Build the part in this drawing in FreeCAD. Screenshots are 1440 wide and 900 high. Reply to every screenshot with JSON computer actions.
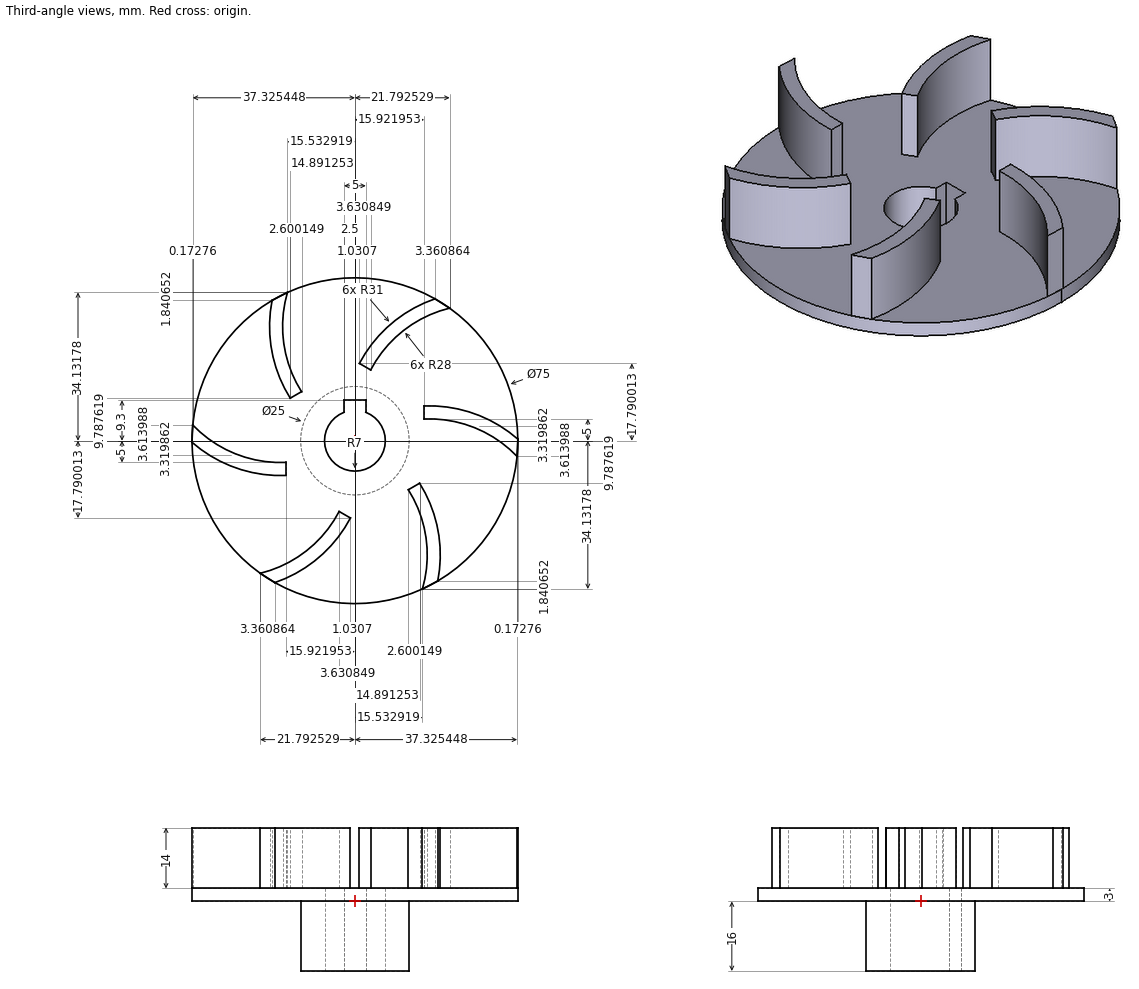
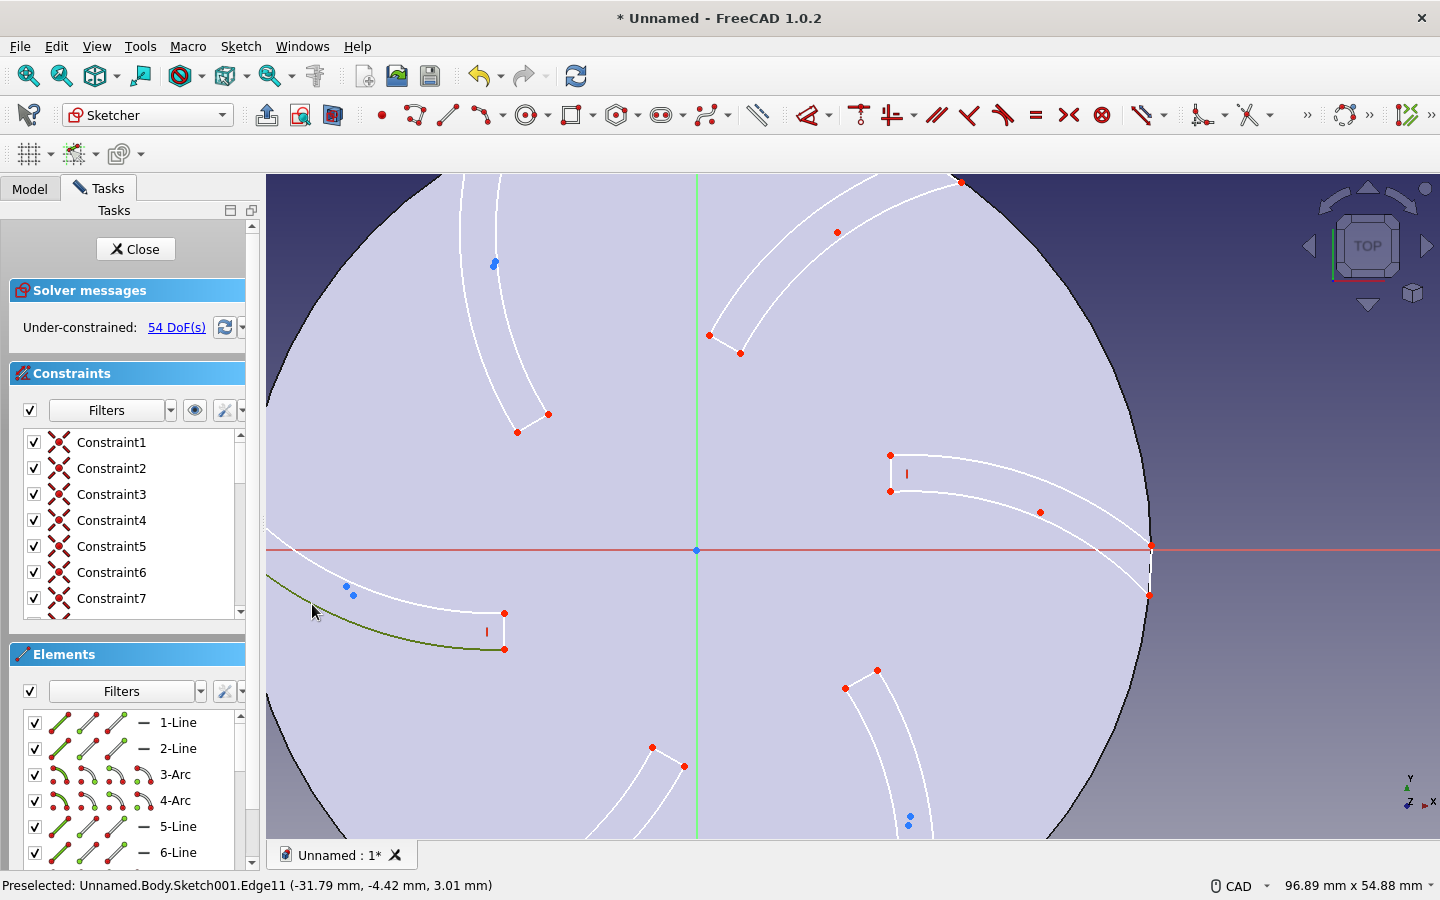
{"action": "scroll", "coordinate": [311, 561], "scroll_direction": "up", "scroll_amount": 2}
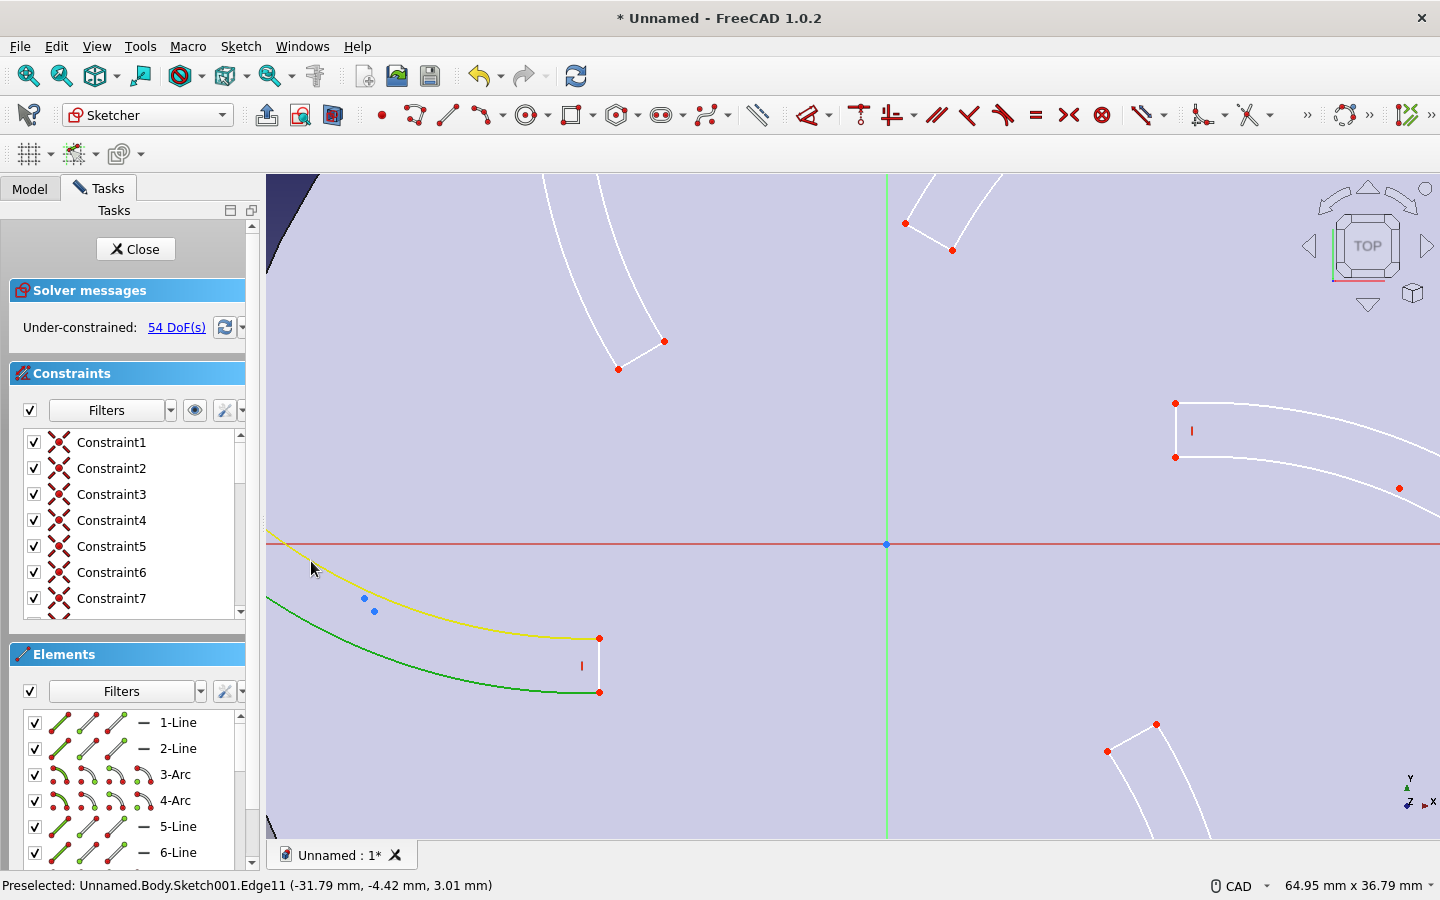
{"action": "left_click", "coordinate": [311, 561]}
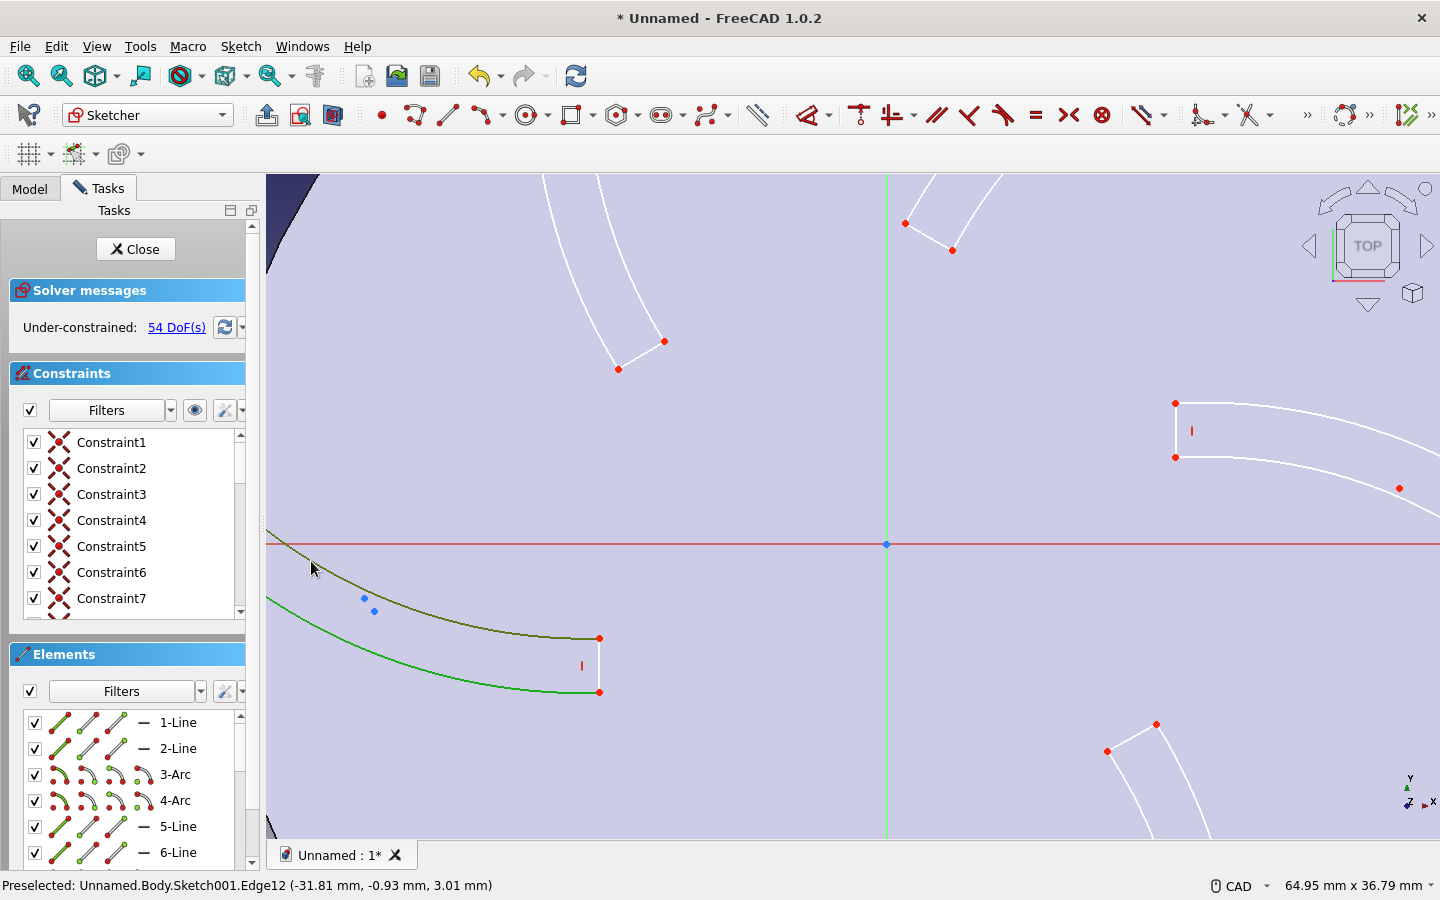
{"action": "left_click", "coordinate": [859, 116]}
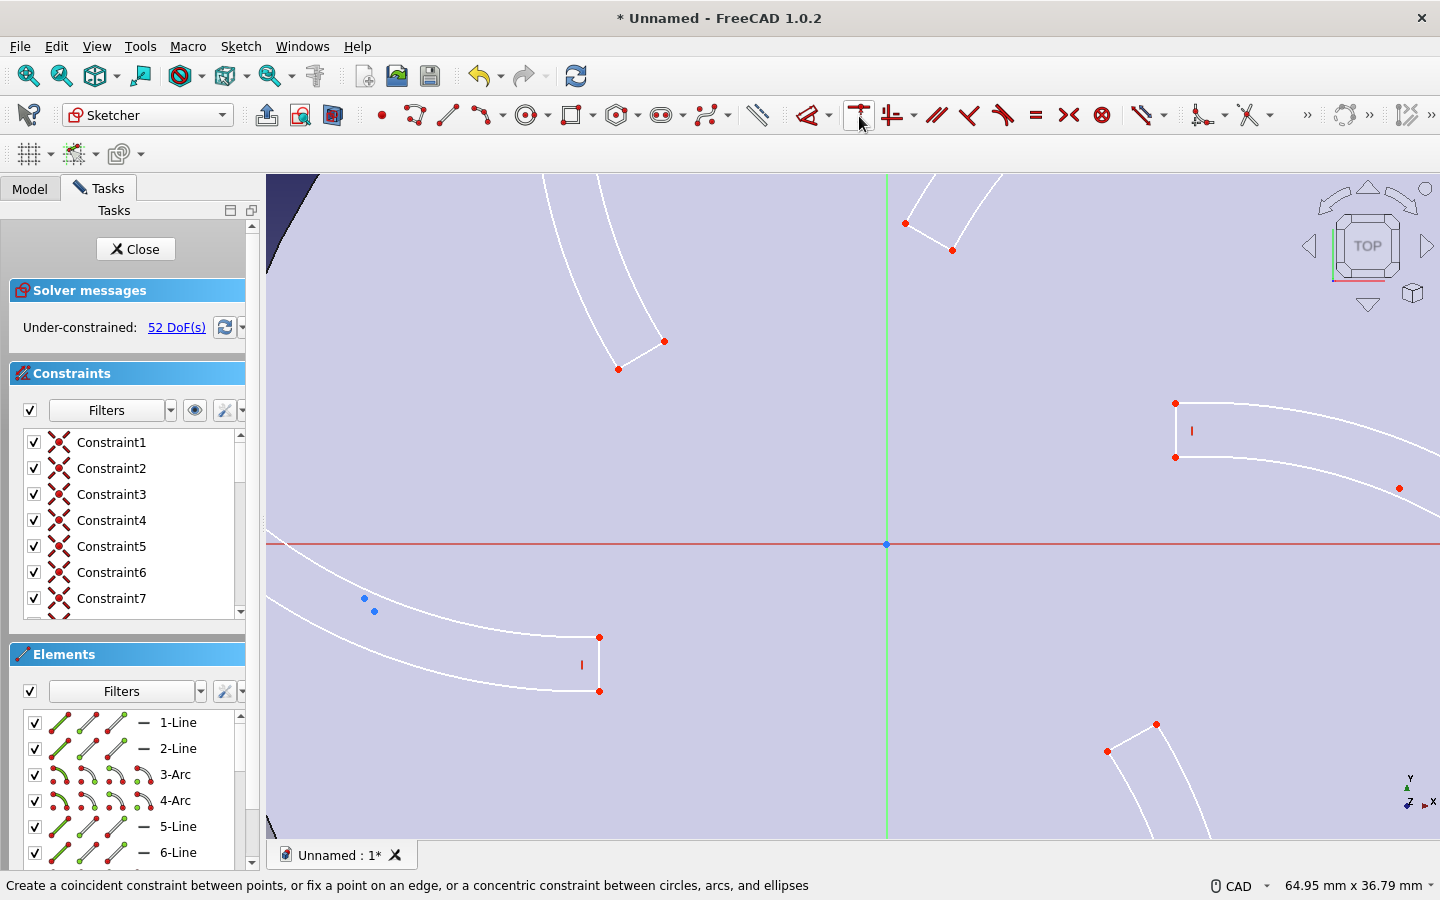
{"action": "scroll", "coordinate": [725, 484], "scroll_direction": "down", "scroll_amount": 5}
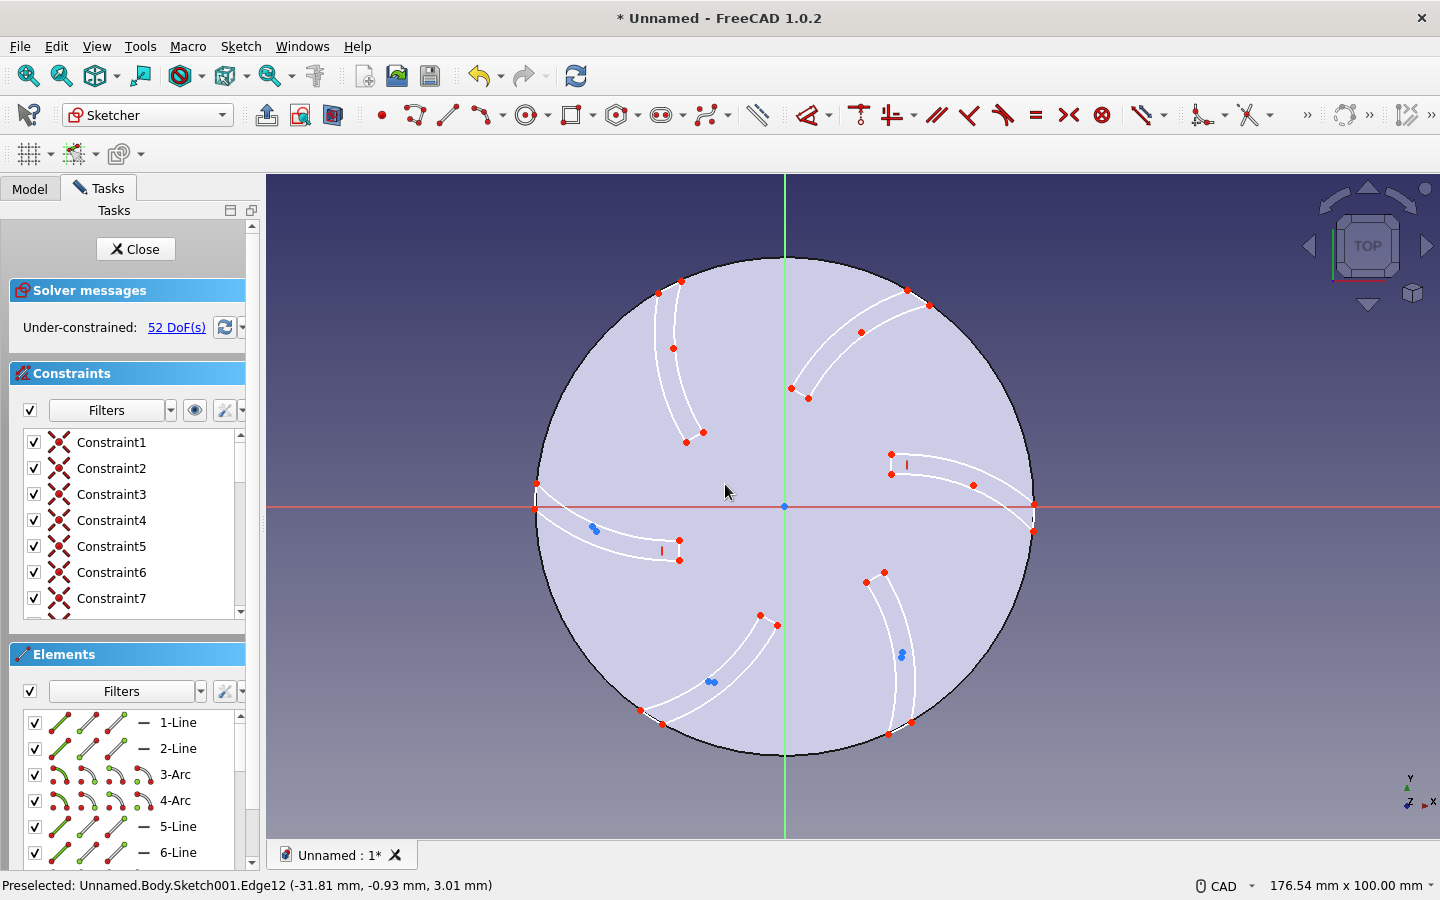
{"action": "left_click", "coordinate": [704, 704]}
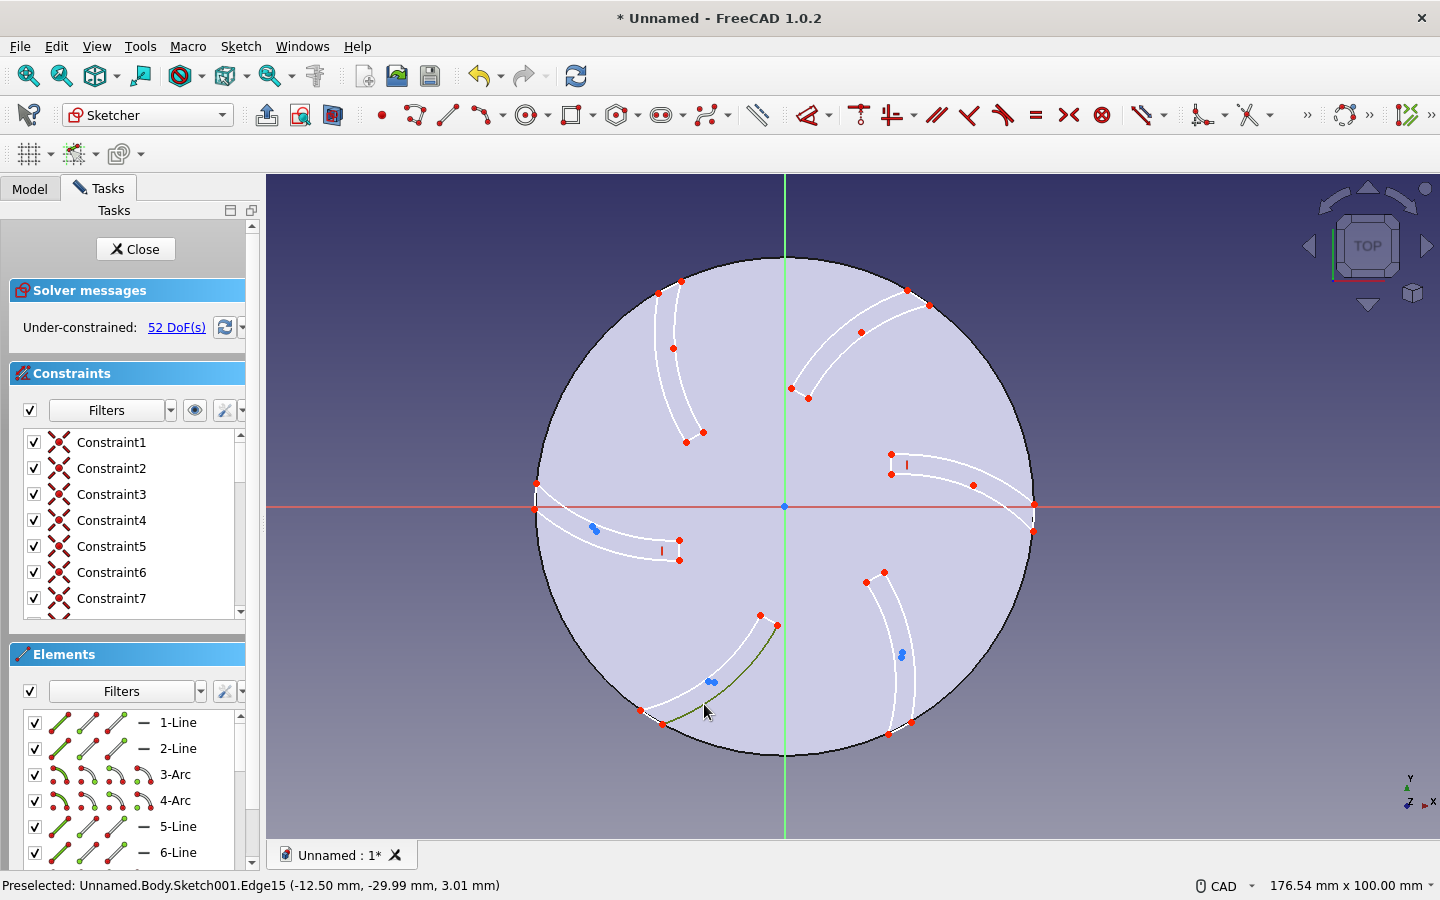
{"action": "left_click", "coordinate": [684, 693]}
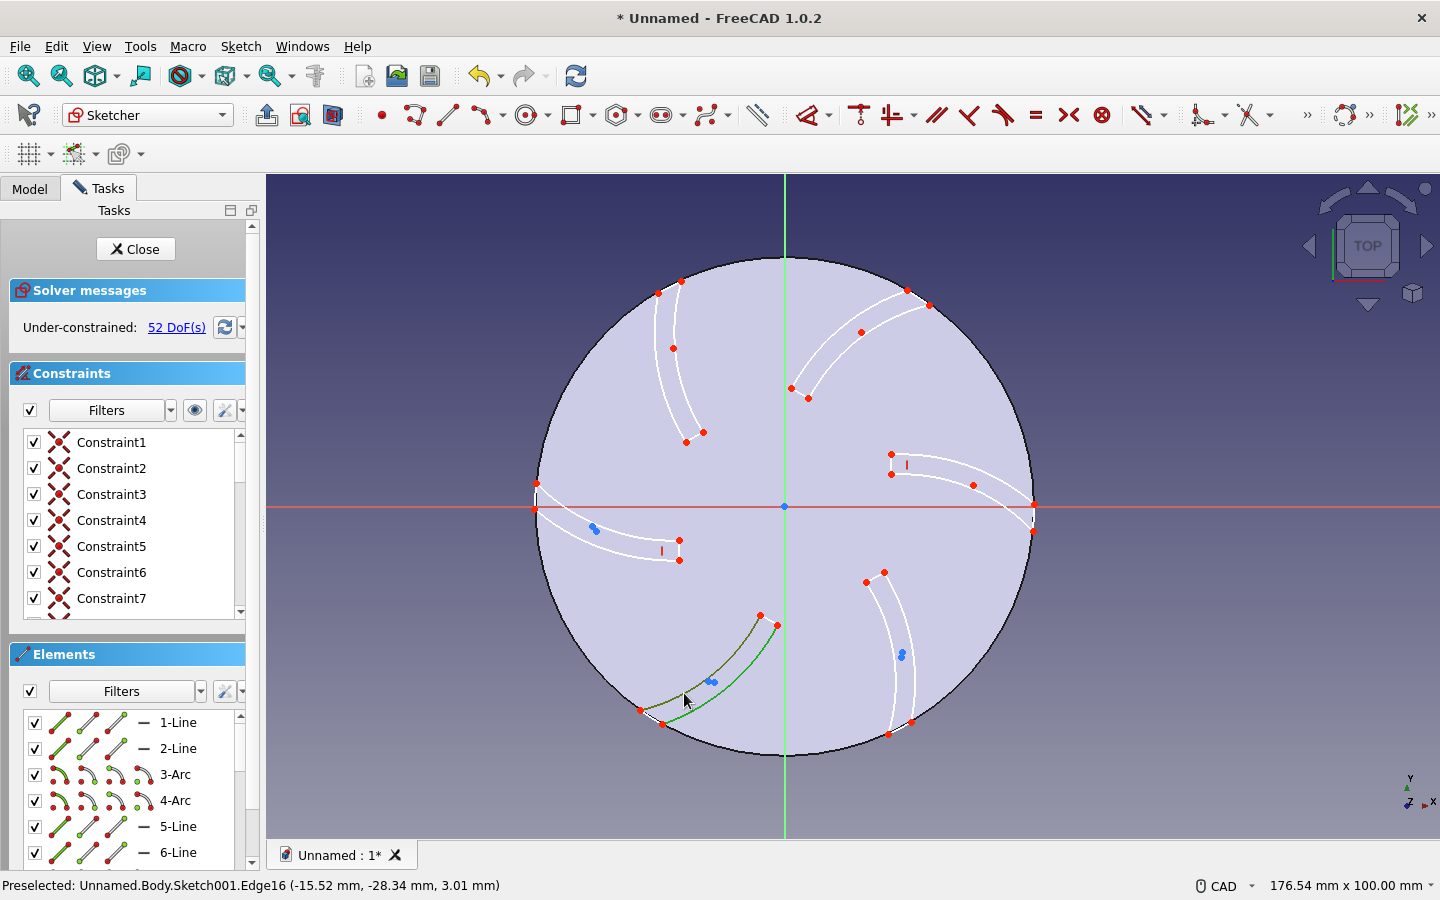
{"action": "left_click", "coordinate": [859, 116]}